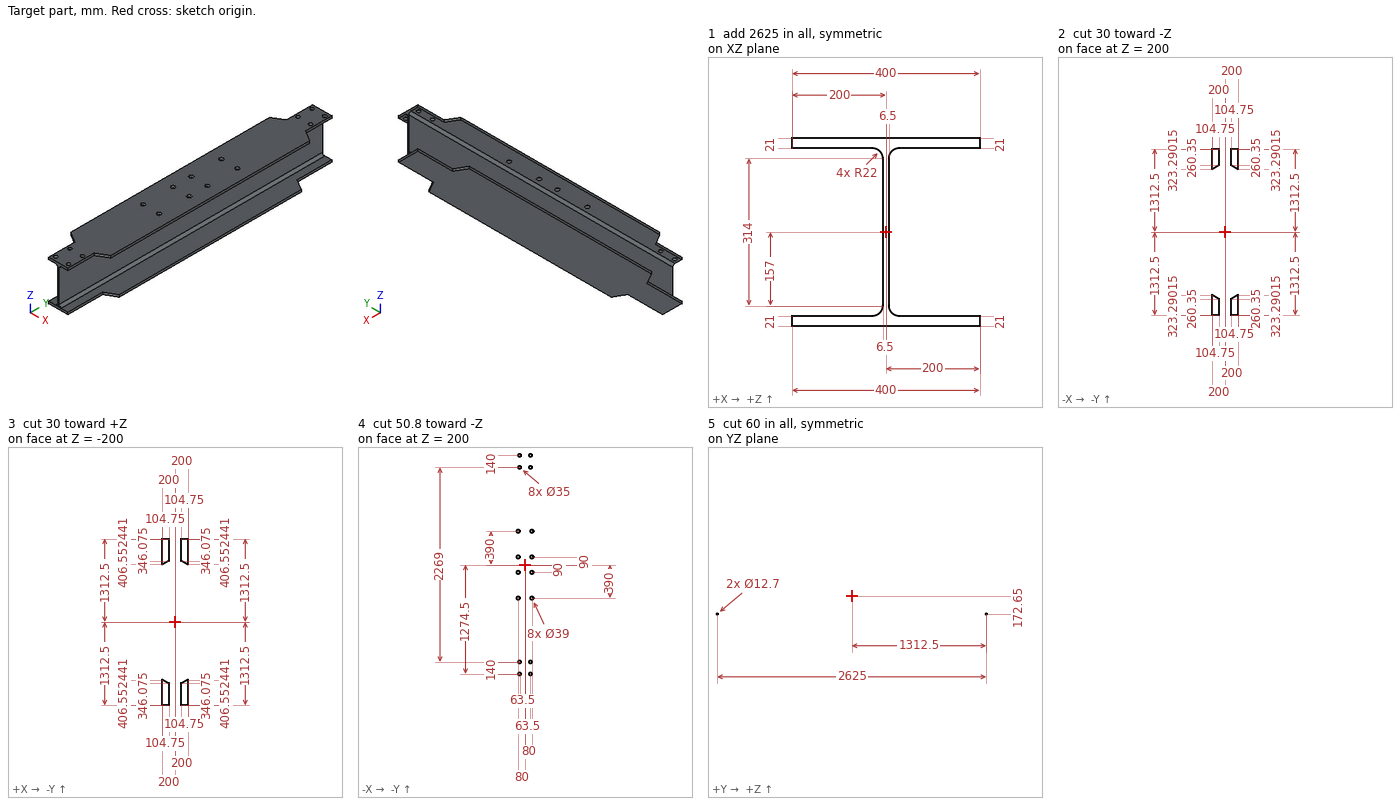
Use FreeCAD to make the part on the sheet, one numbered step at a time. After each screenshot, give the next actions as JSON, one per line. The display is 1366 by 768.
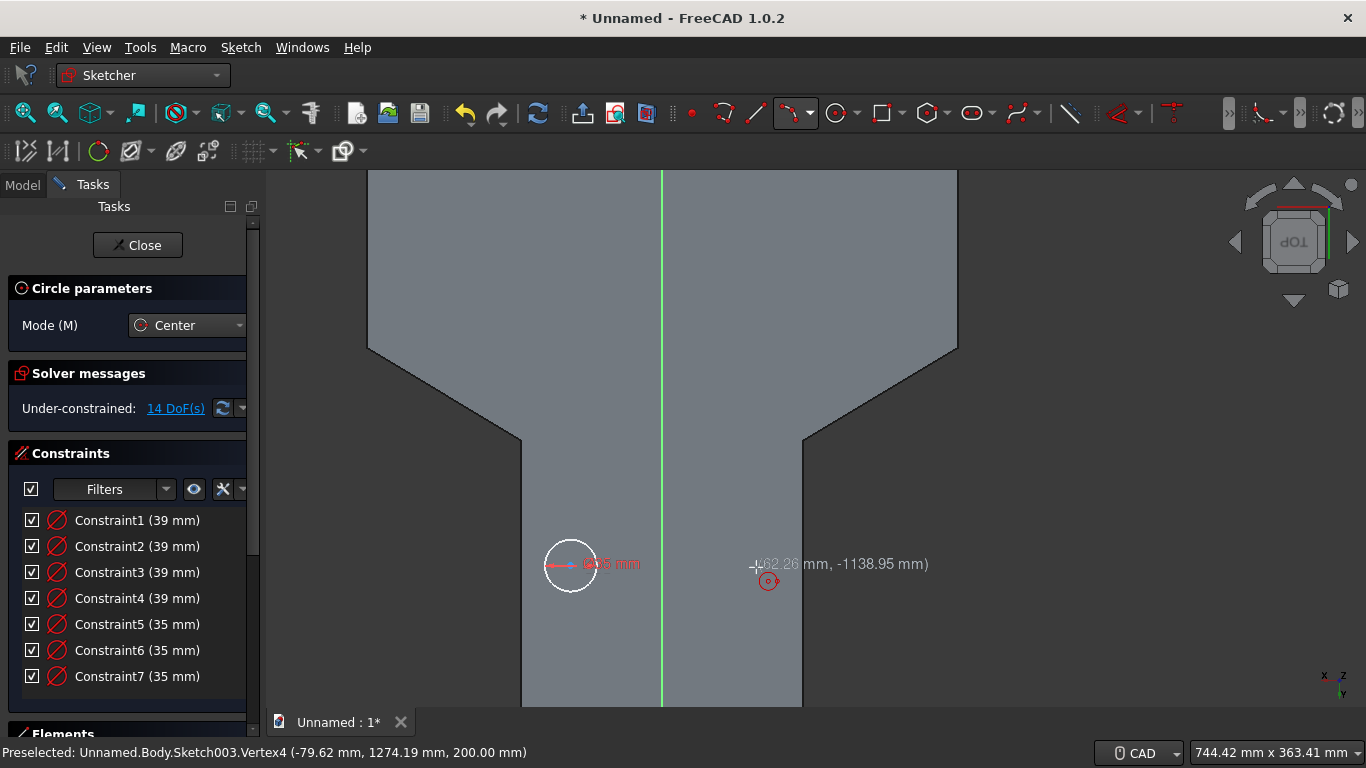
{"action": "scroll", "coordinate": [756, 593], "scroll_direction": "down", "scroll_amount": 12}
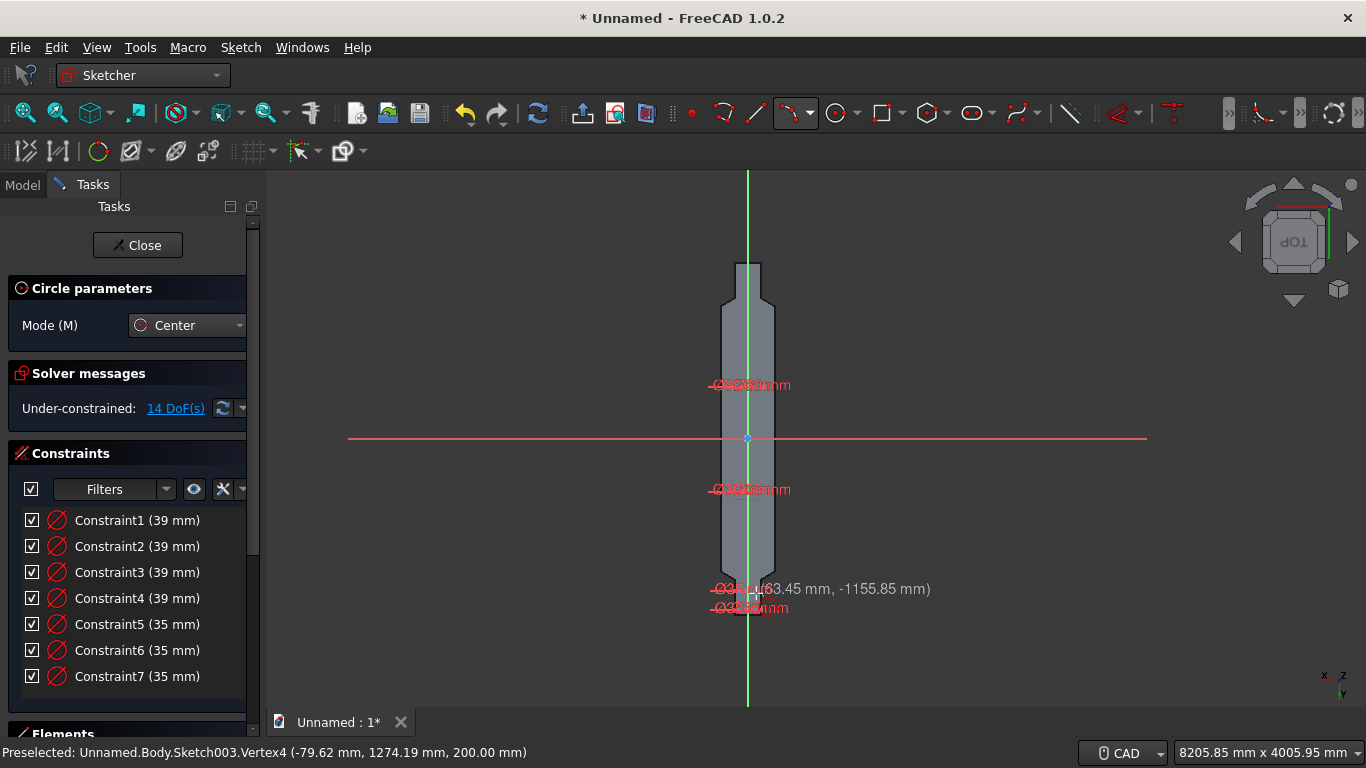
{"action": "scroll", "coordinate": [756, 591], "scroll_direction": "up", "scroll_amount": 4}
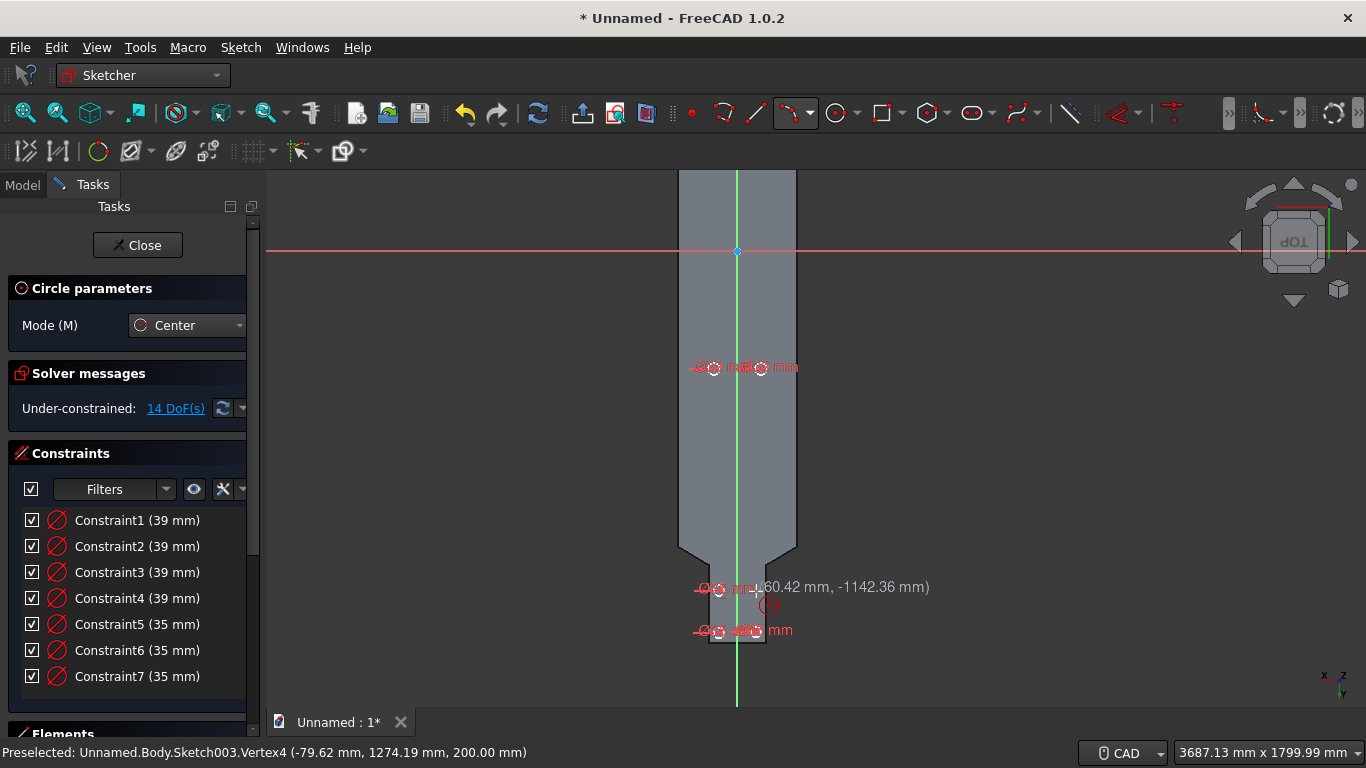
{"action": "left_click", "coordinate": [756, 590]}
{"action": "mouse_move", "coordinate": [760, 586]}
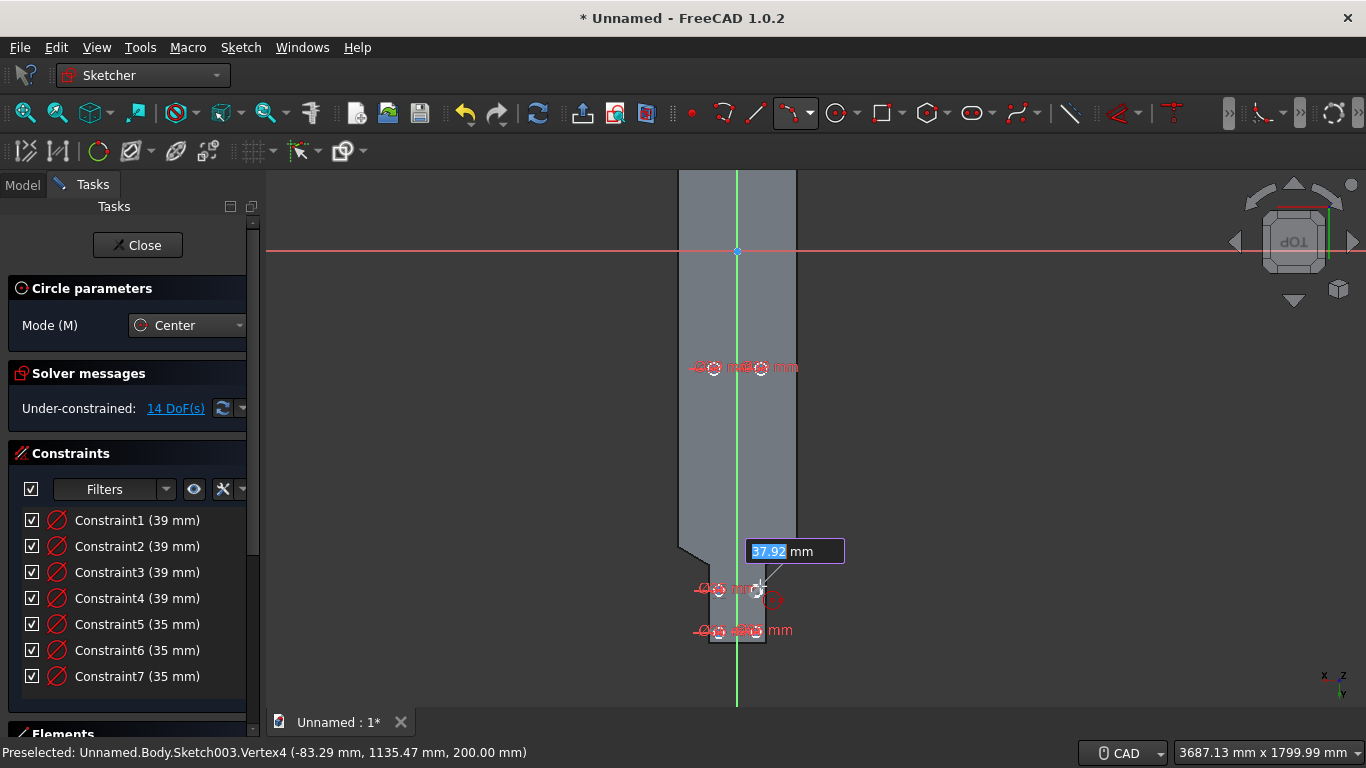
{"action": "type", "text": "35"}
{"action": "key", "text": "Return"}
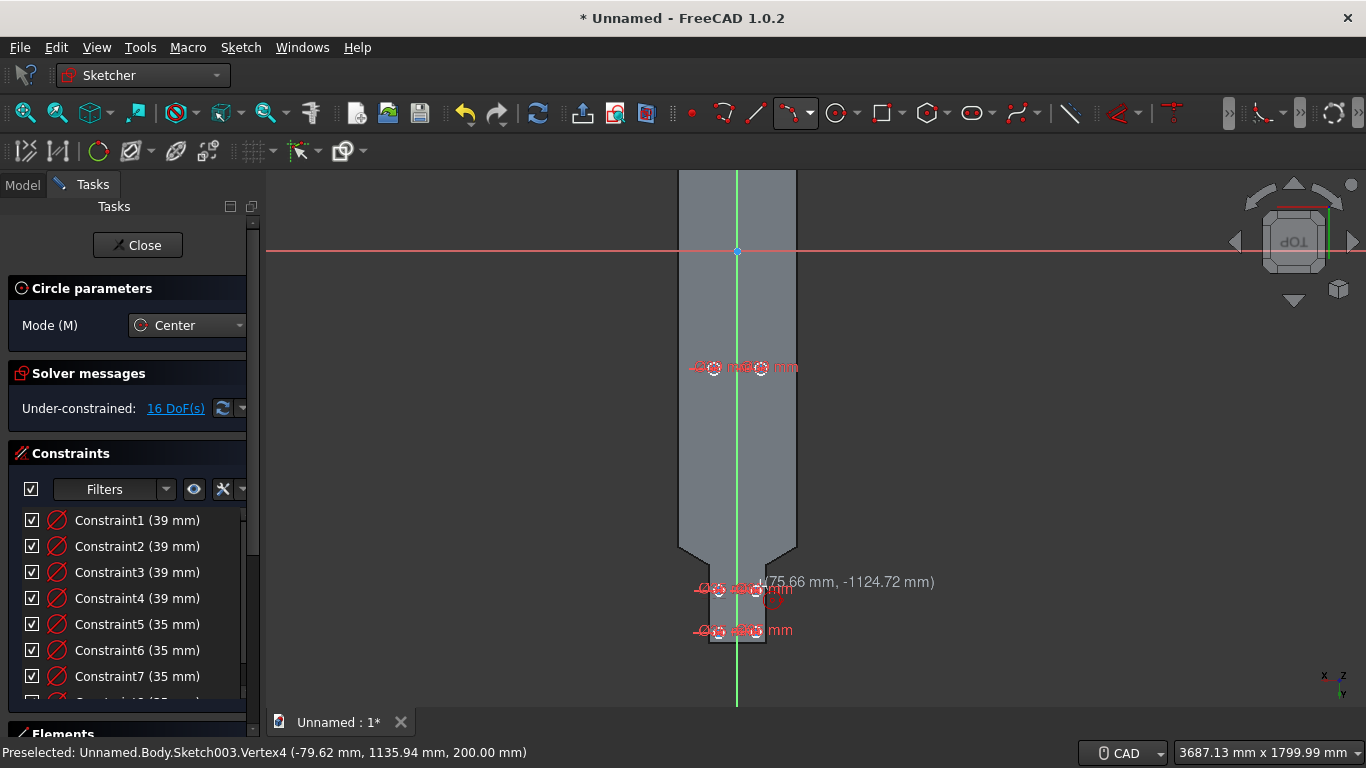
{"action": "scroll", "coordinate": [756, 591], "scroll_direction": "down", "scroll_amount": 4}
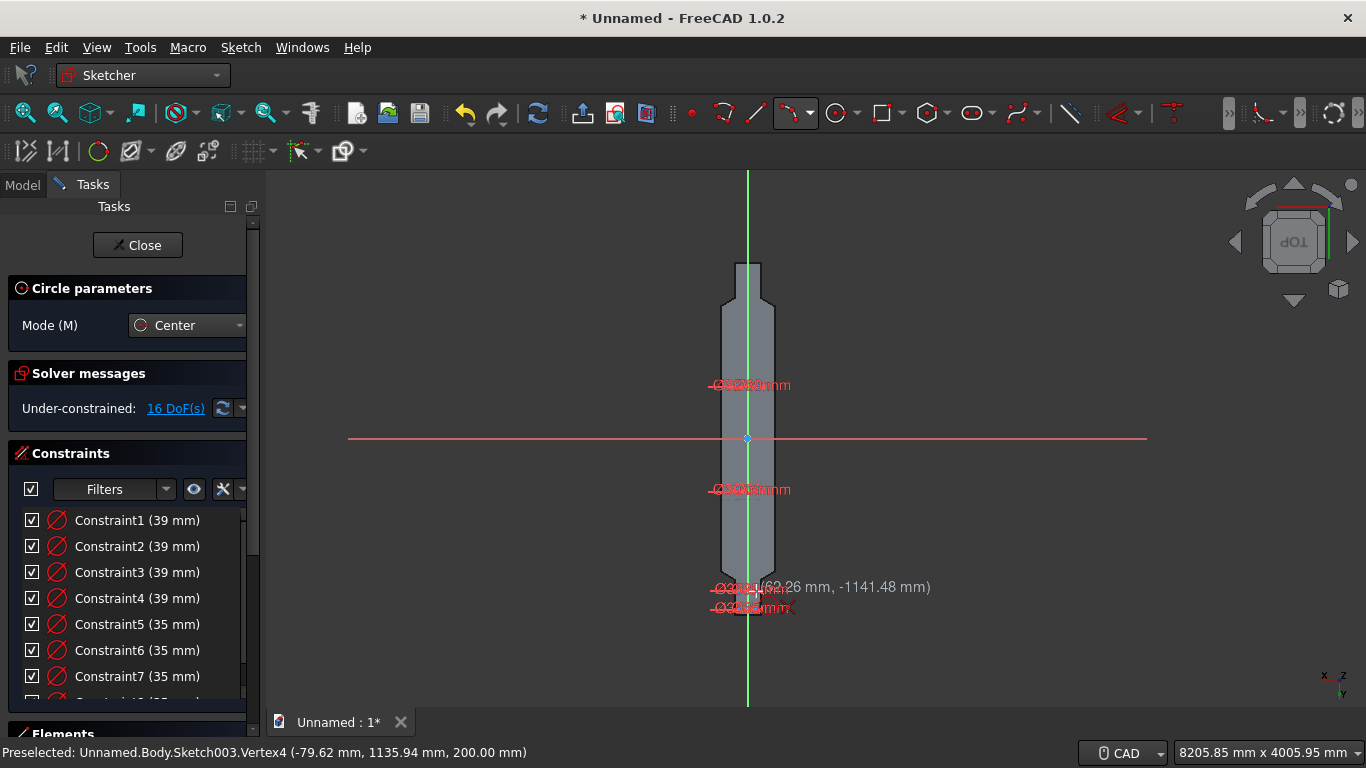
{"action": "scroll", "coordinate": [739, 287], "scroll_direction": "up", "scroll_amount": 12}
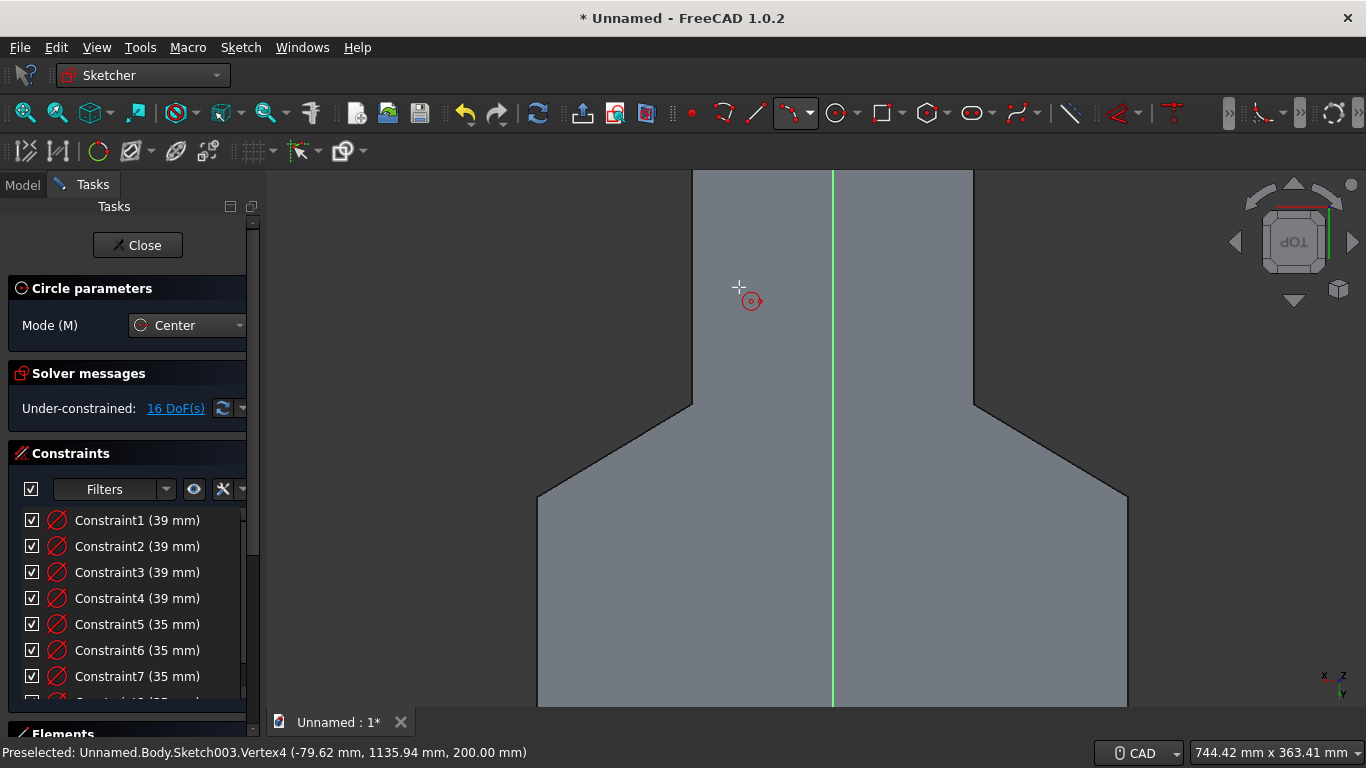
{"action": "scroll", "coordinate": [739, 287], "scroll_direction": "down", "scroll_amount": 12}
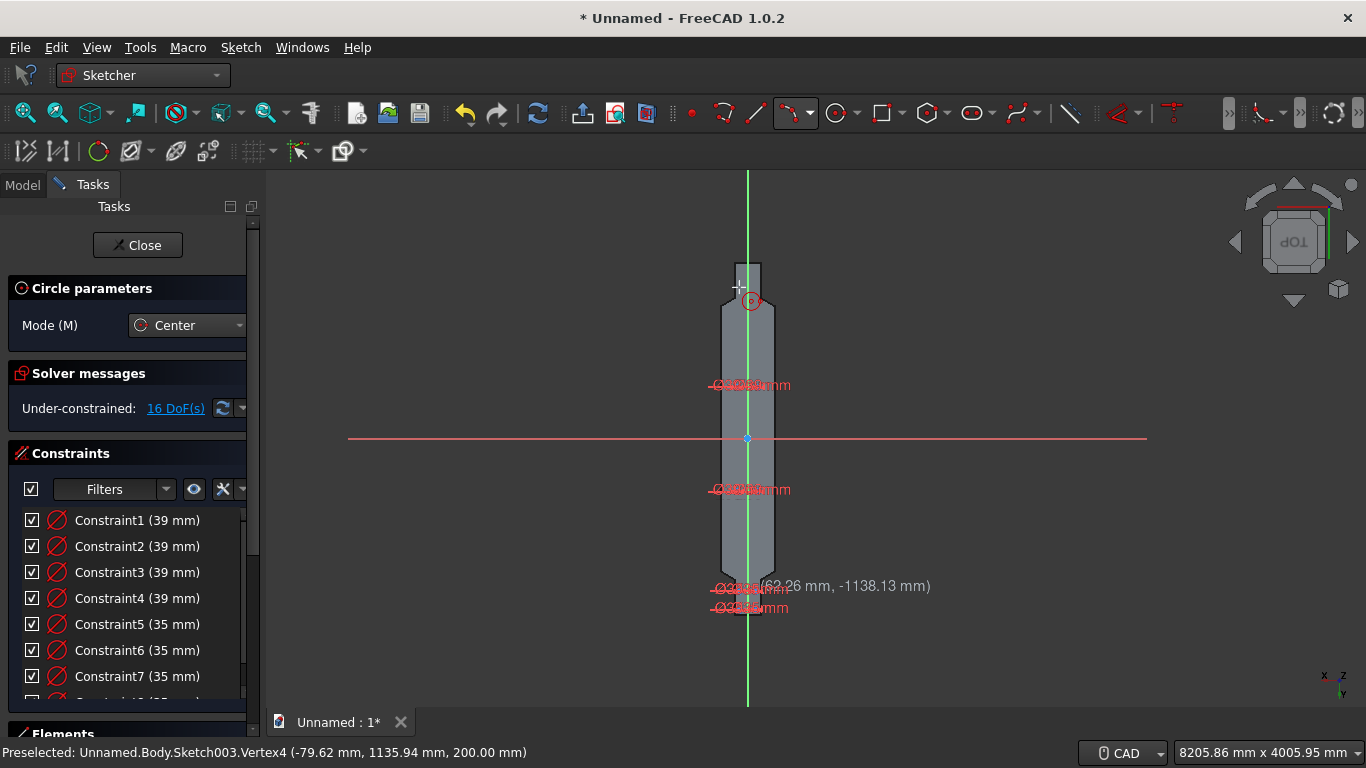
{"action": "scroll", "coordinate": [739, 287], "scroll_direction": "up", "scroll_amount": 4}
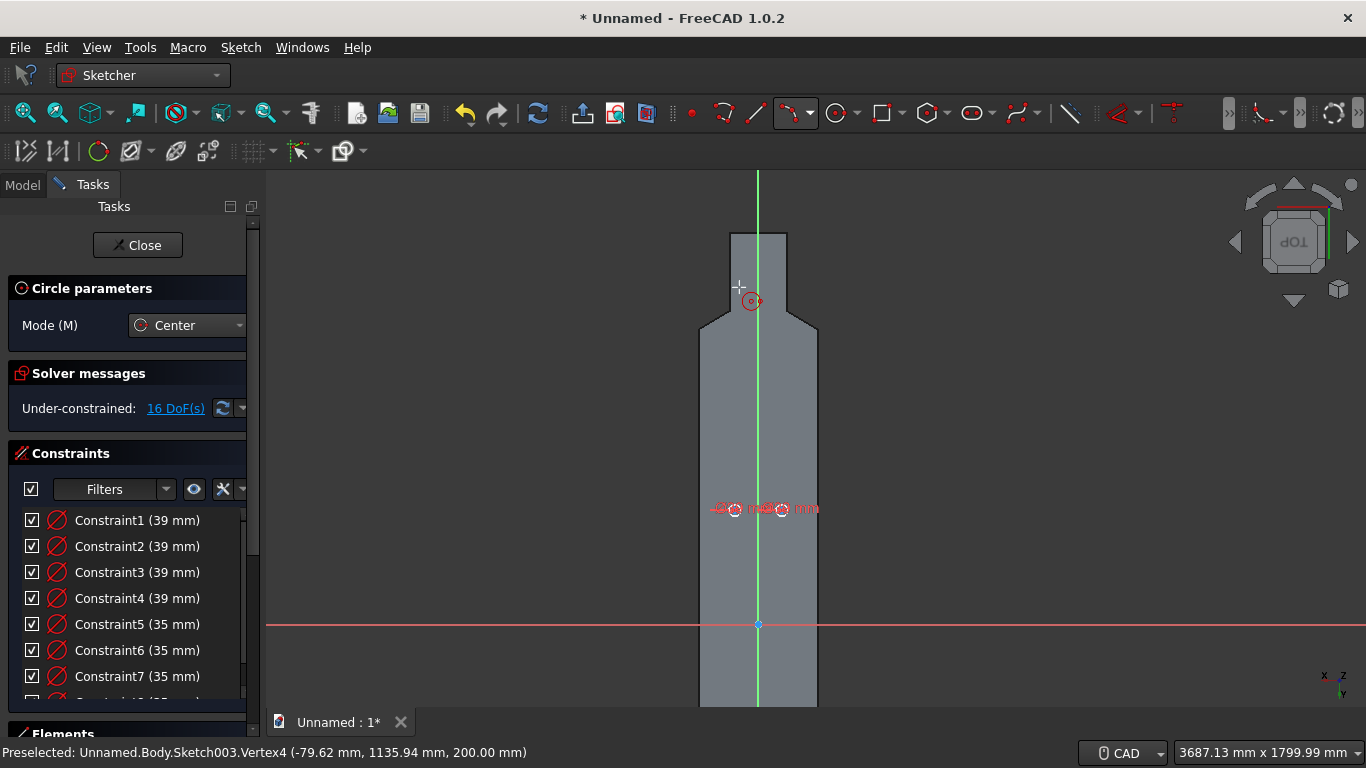
{"action": "left_click", "coordinate": [739, 286]}
{"action": "mouse_move", "coordinate": [743, 283]}